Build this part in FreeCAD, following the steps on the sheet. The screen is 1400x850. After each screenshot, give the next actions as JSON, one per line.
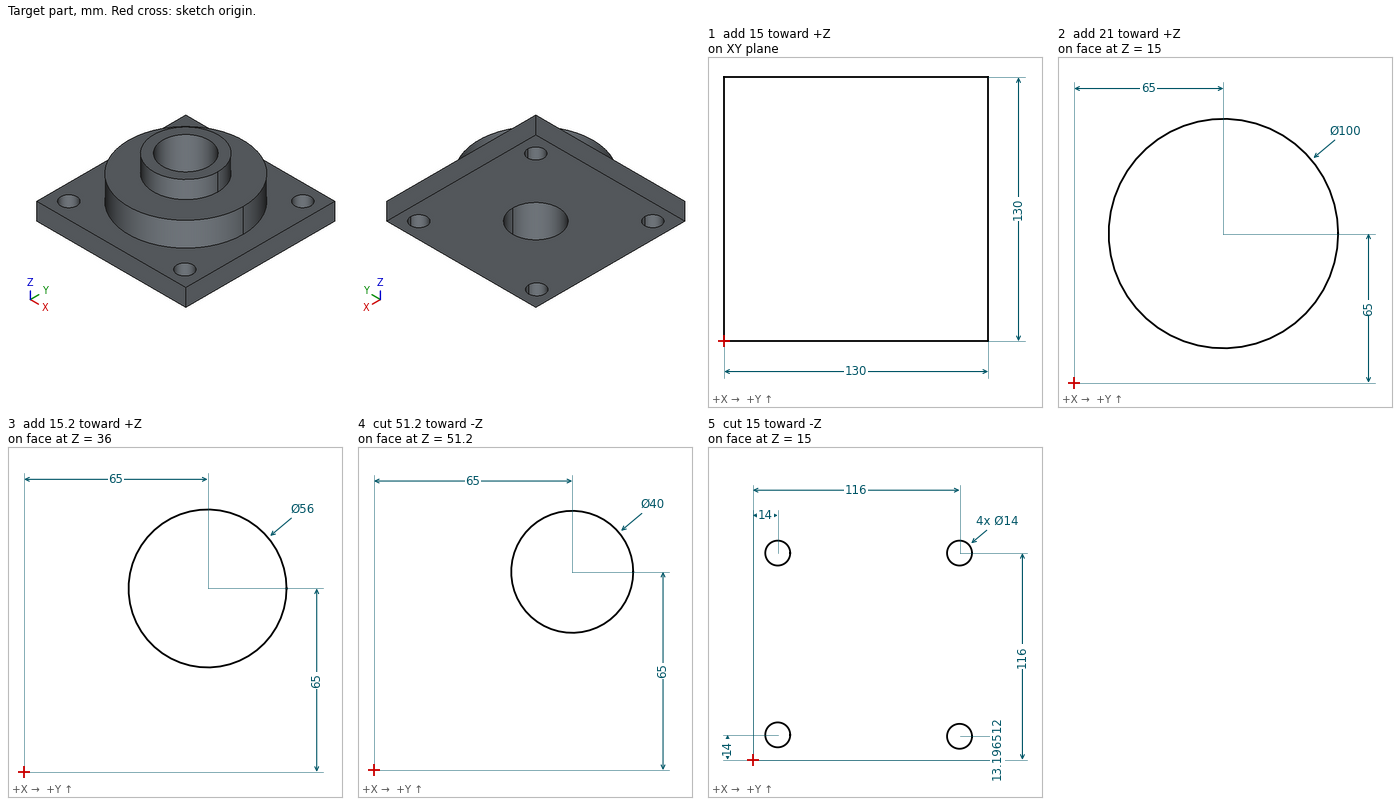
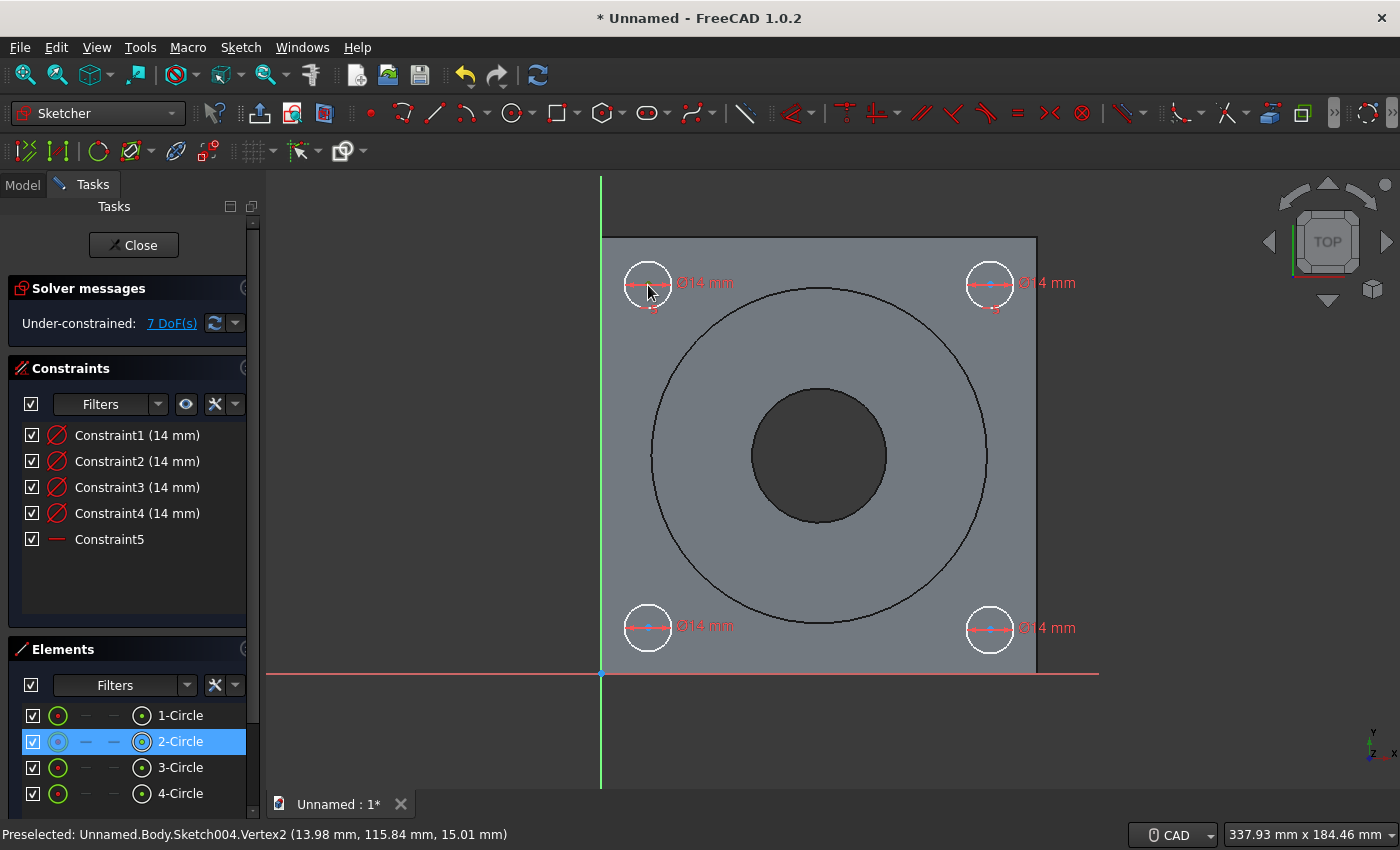
{"action": "left_click", "coordinate": [648, 628]}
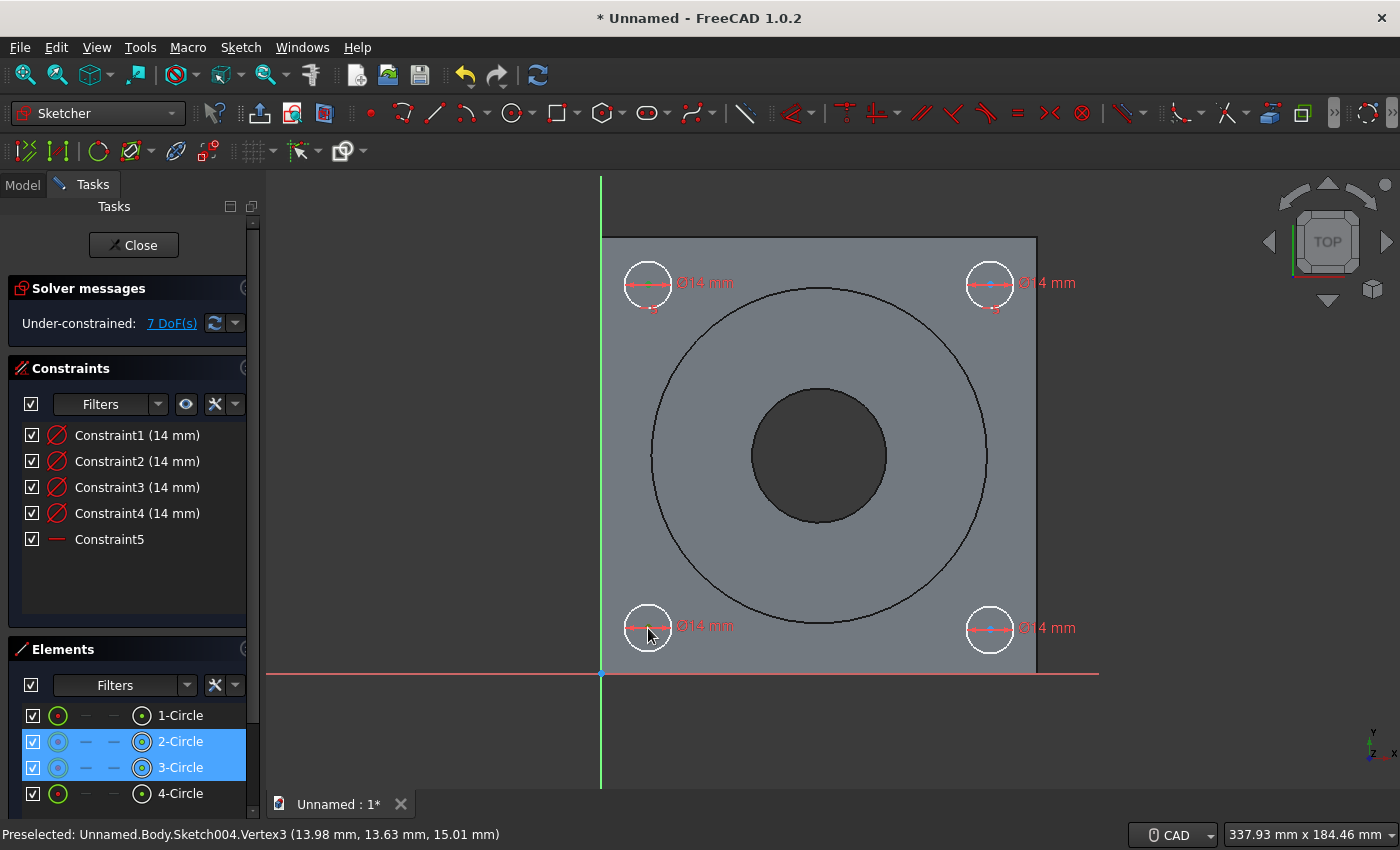
{"action": "key", "text": "v"}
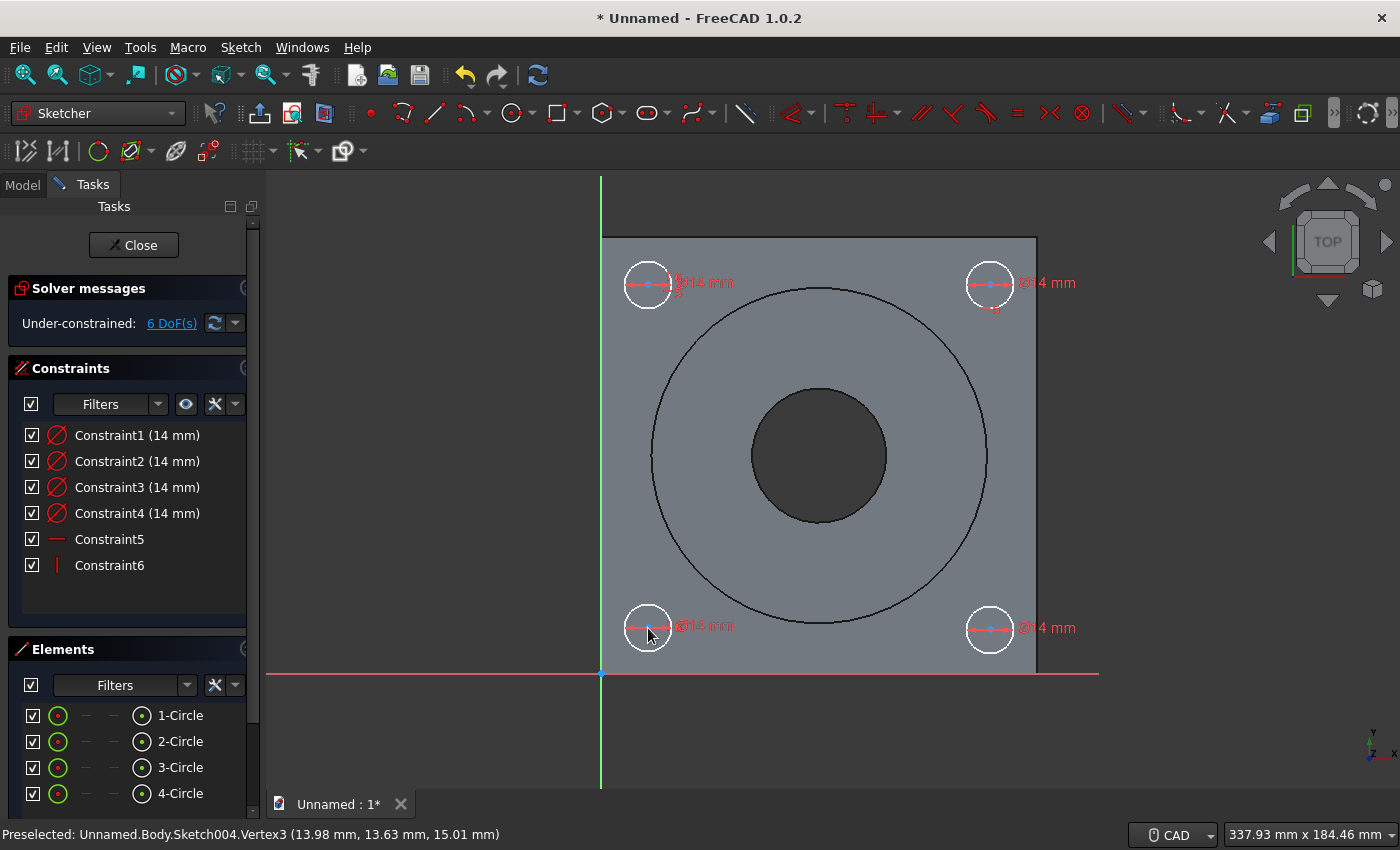
{"action": "left_click", "coordinate": [990, 285]}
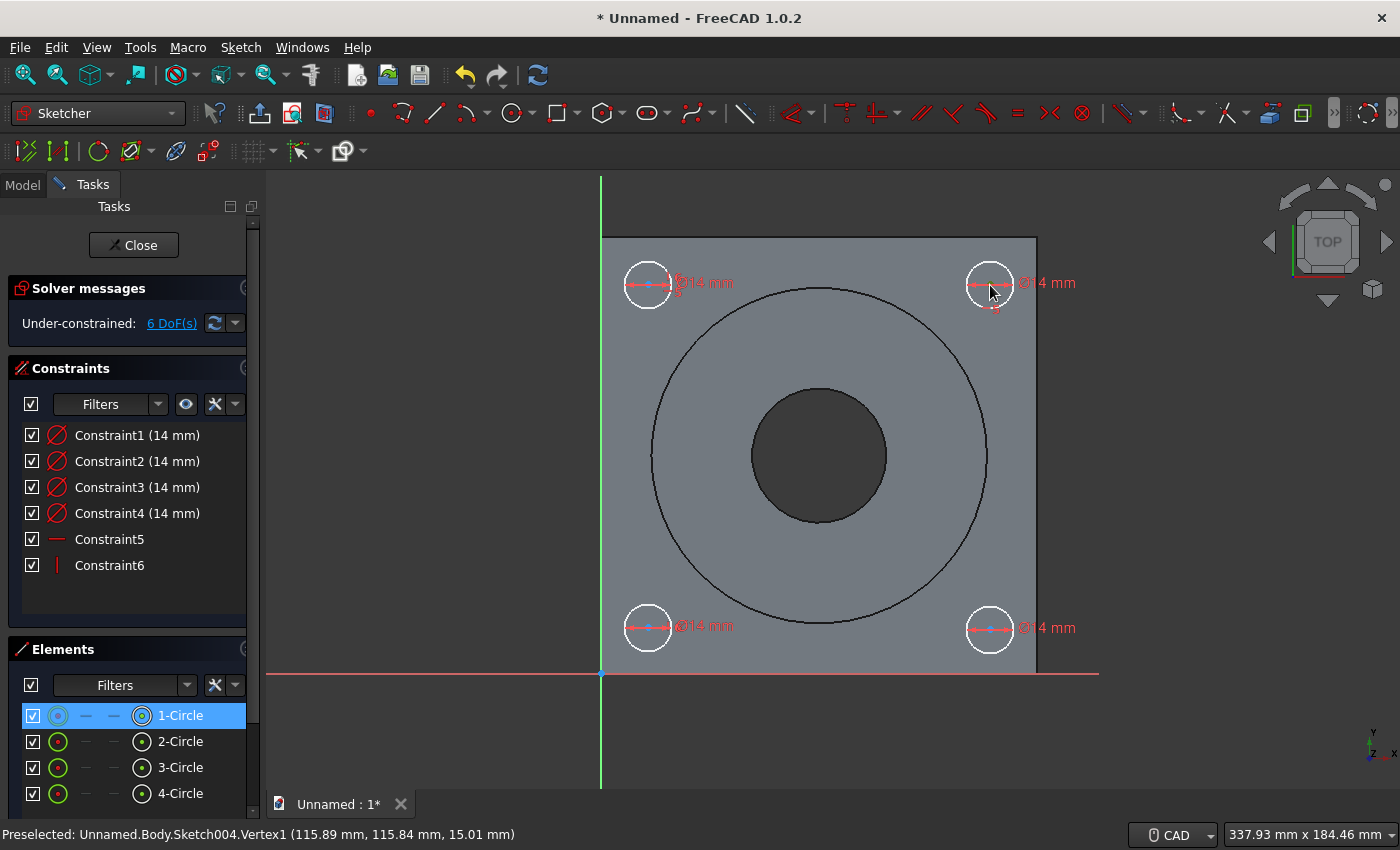
{"action": "left_click", "coordinate": [990, 630]}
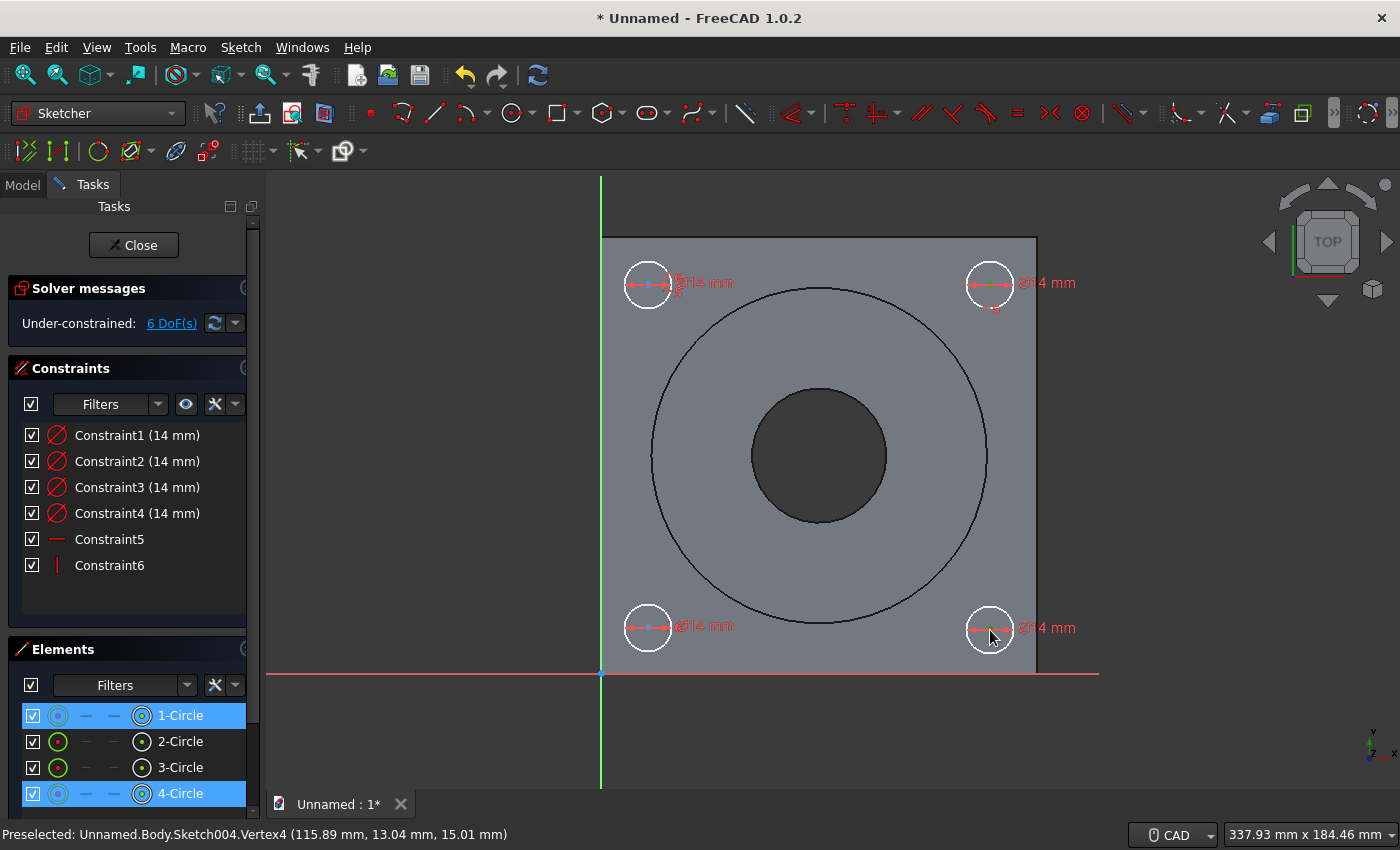
{"action": "key", "text": "v"}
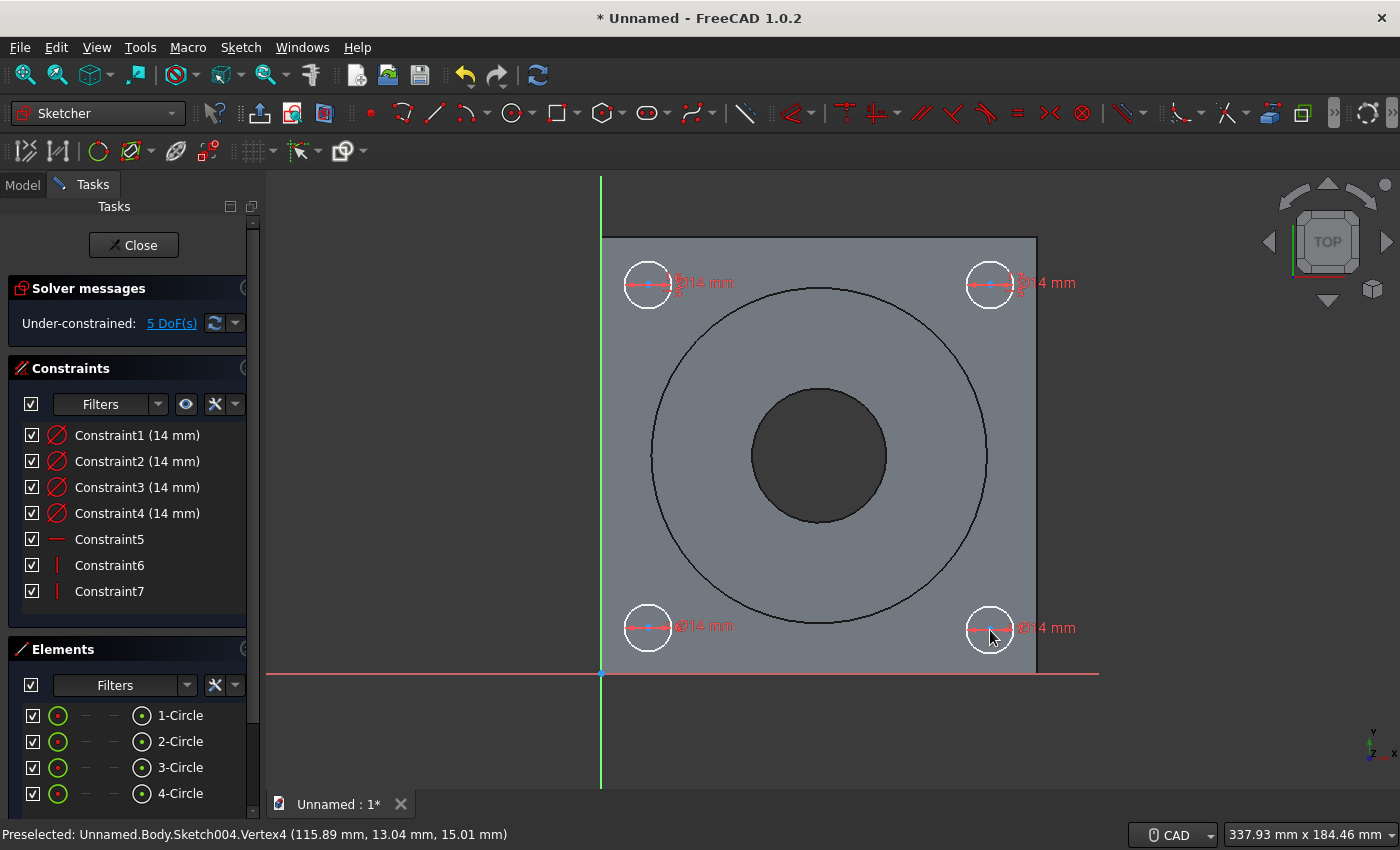
{"action": "key", "text": "d"}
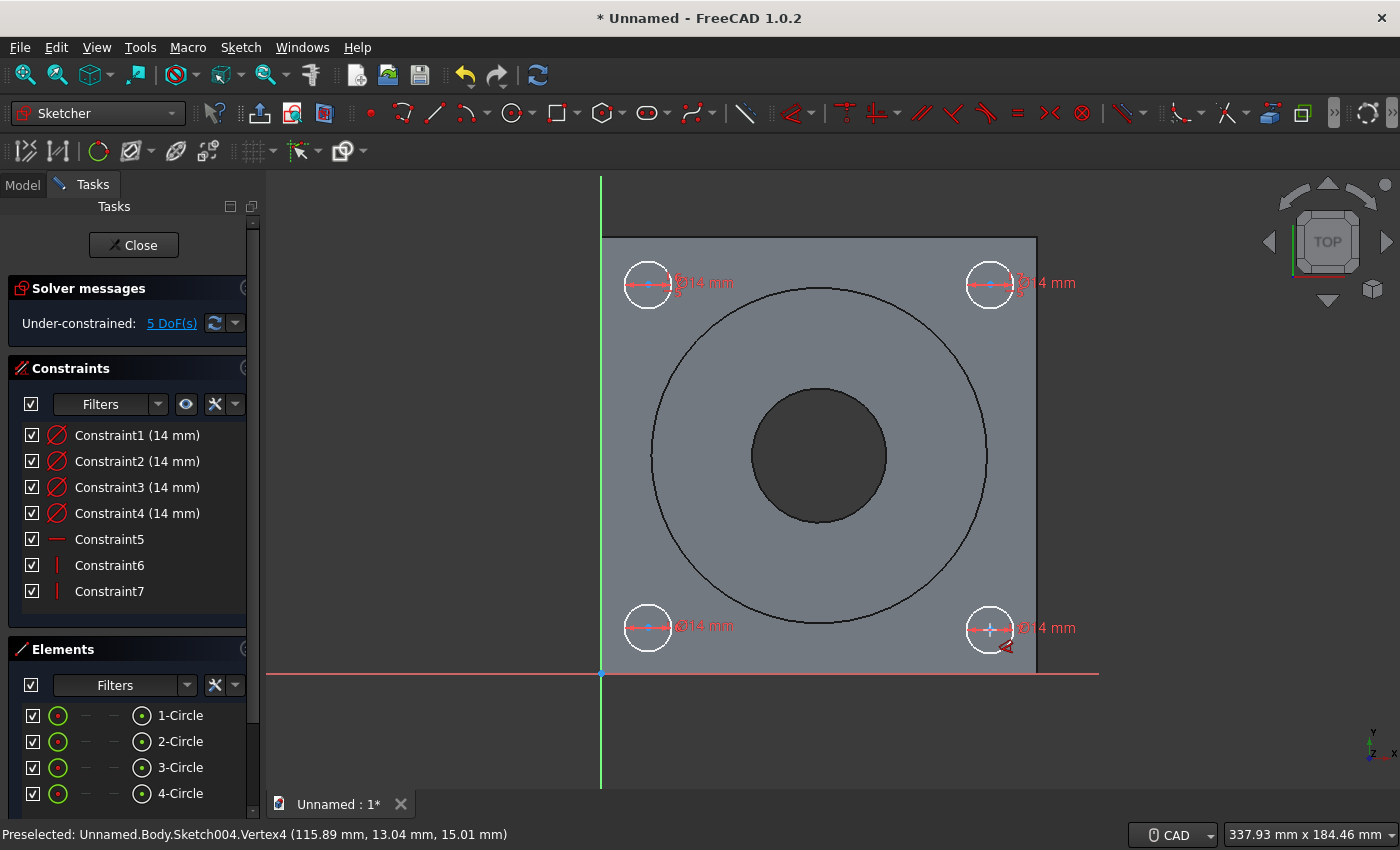
{"action": "left_click", "coordinate": [648, 285]}
{"action": "left_click", "coordinate": [625, 708]}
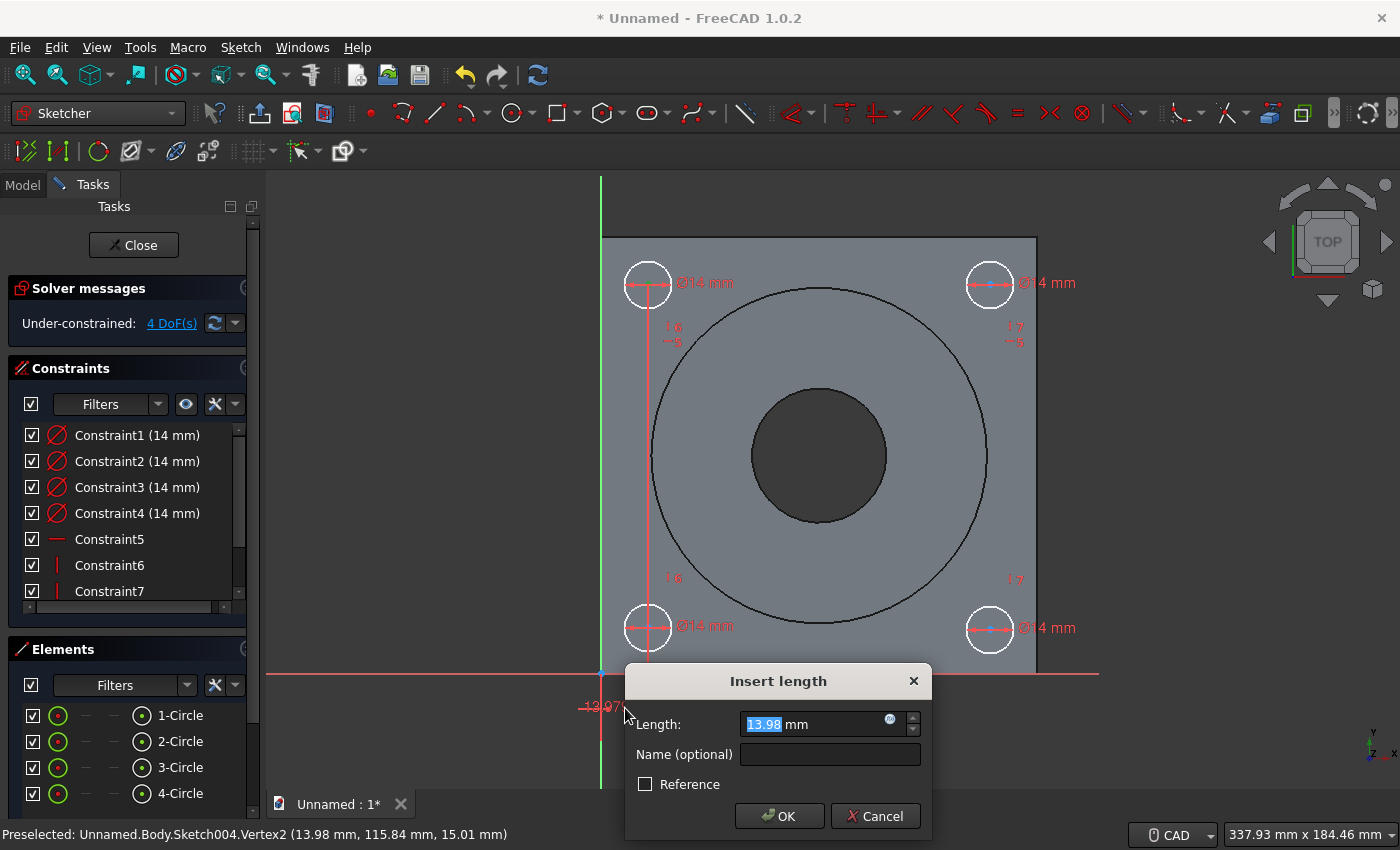
{"action": "type", "text": "14"}
{"action": "key", "text": "Return"}